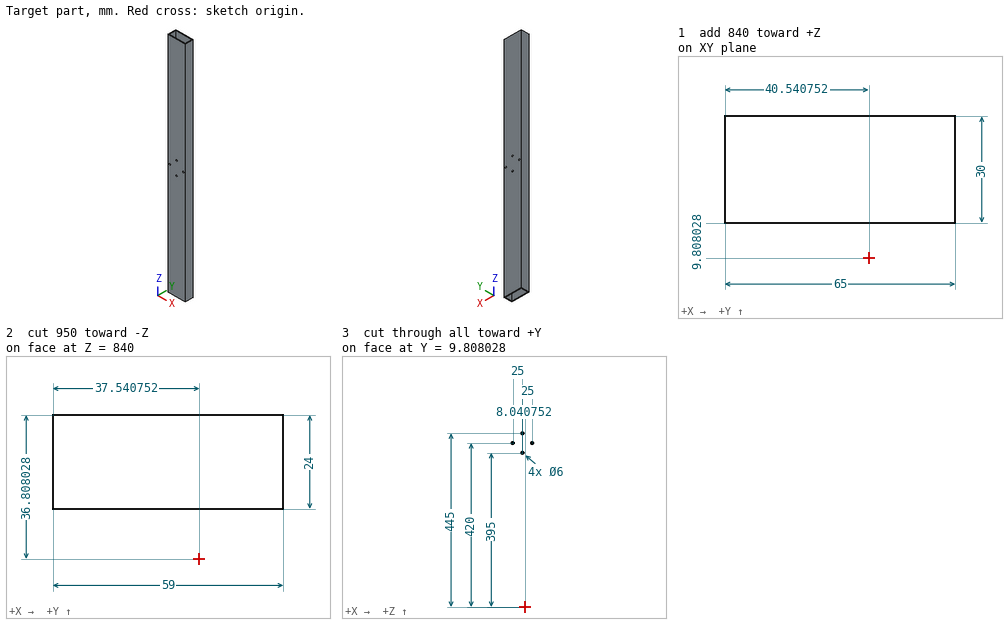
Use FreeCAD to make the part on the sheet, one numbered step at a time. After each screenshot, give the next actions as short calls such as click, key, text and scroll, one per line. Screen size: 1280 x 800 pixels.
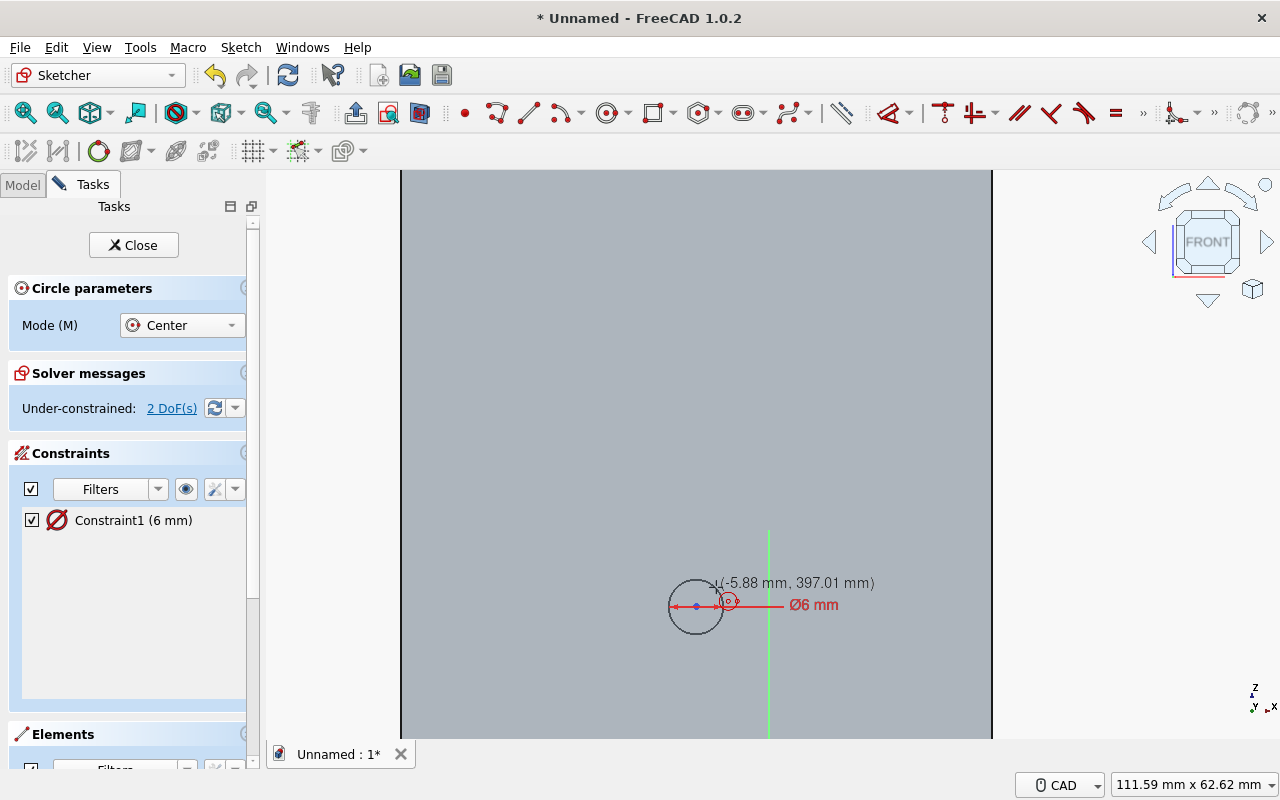
click(469, 379)
move(488, 360)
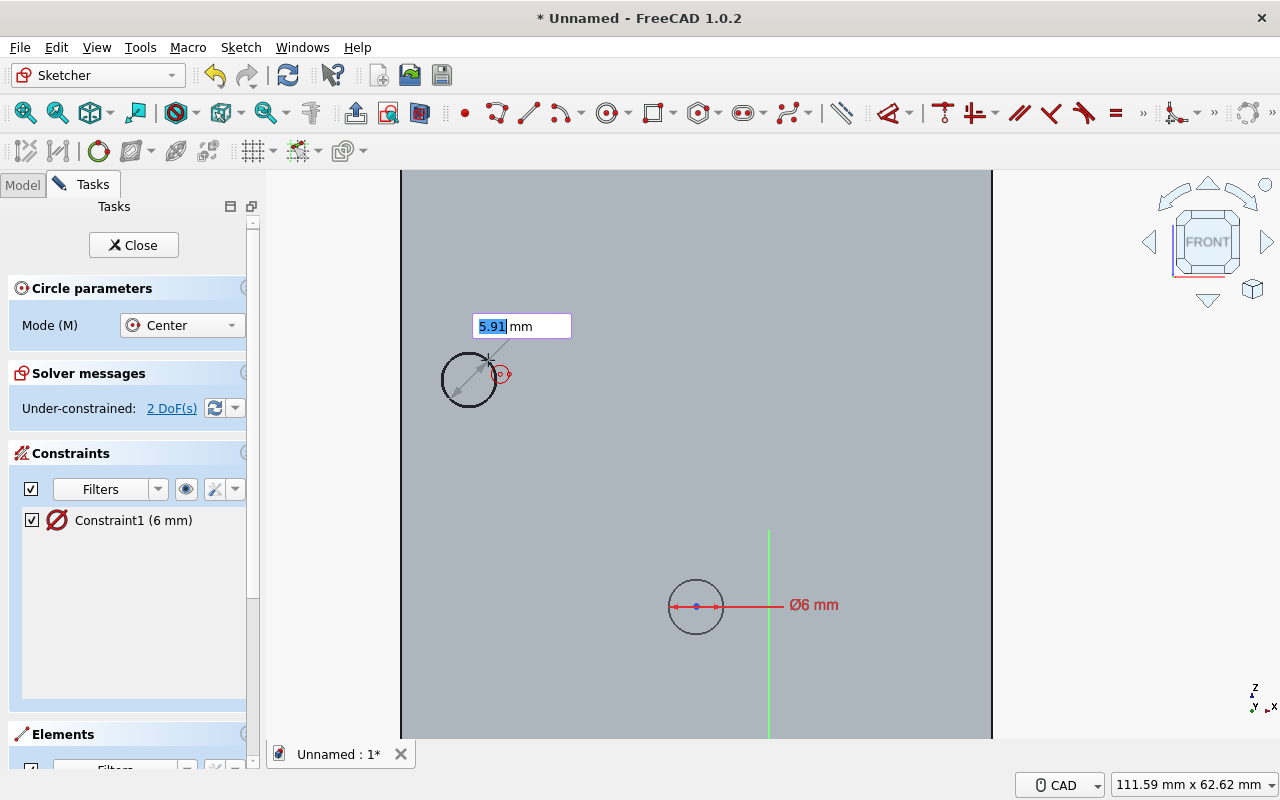
text(6)
key(Return)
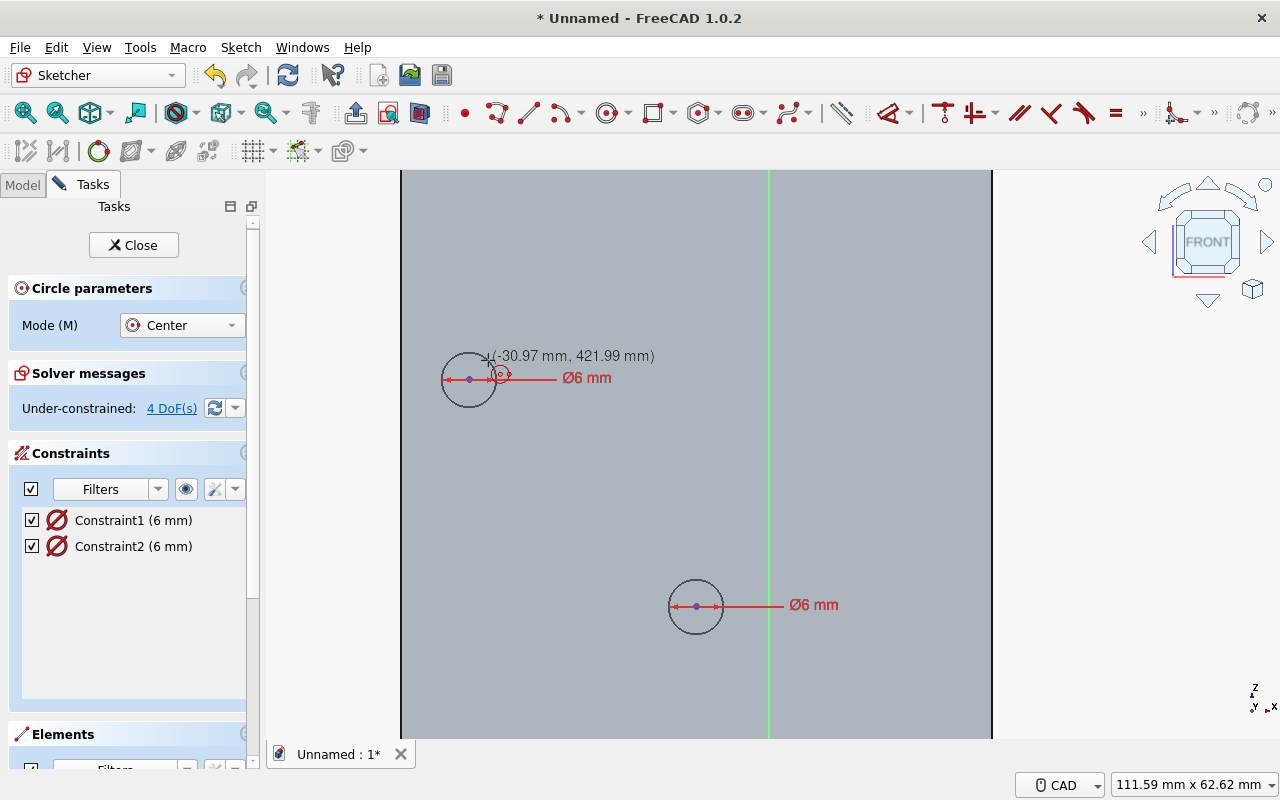
scroll(721, 608, down, 2)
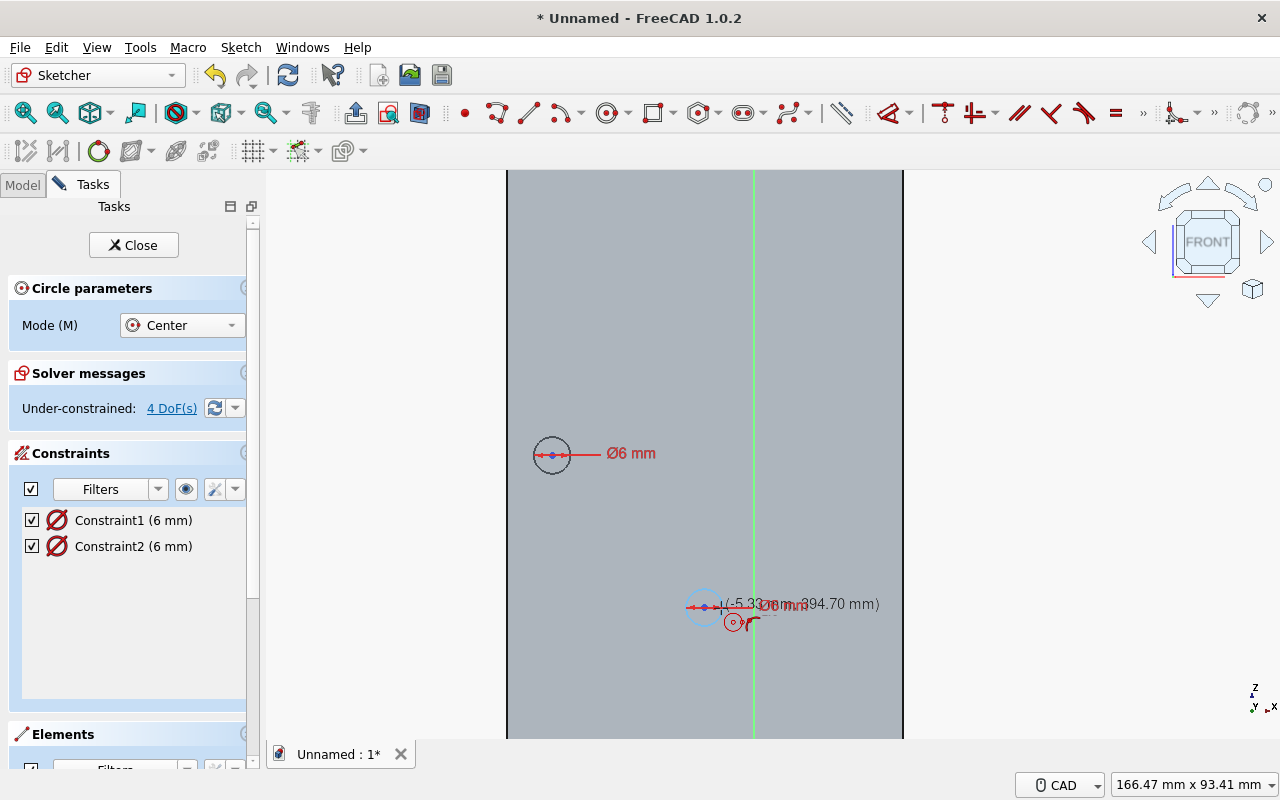
scroll(705, 303, up, 2)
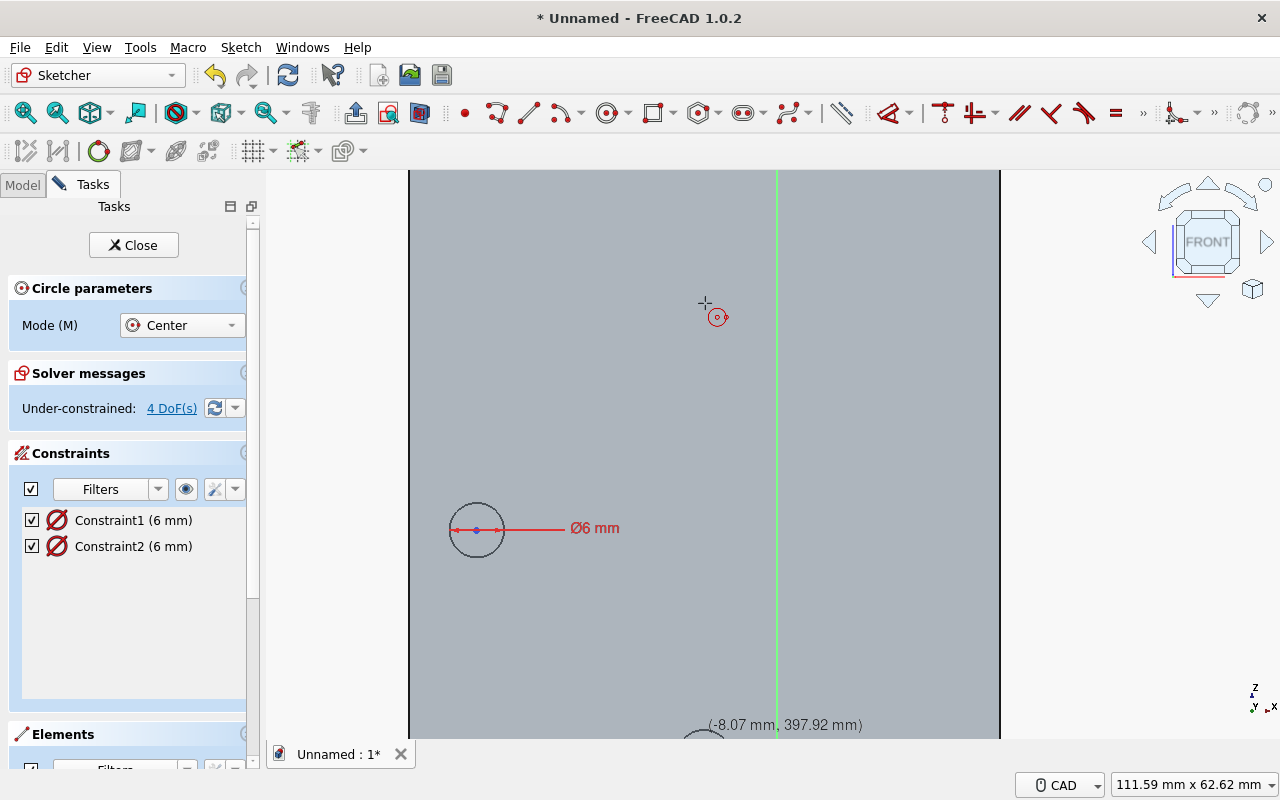
click(704, 302)
move(723, 283)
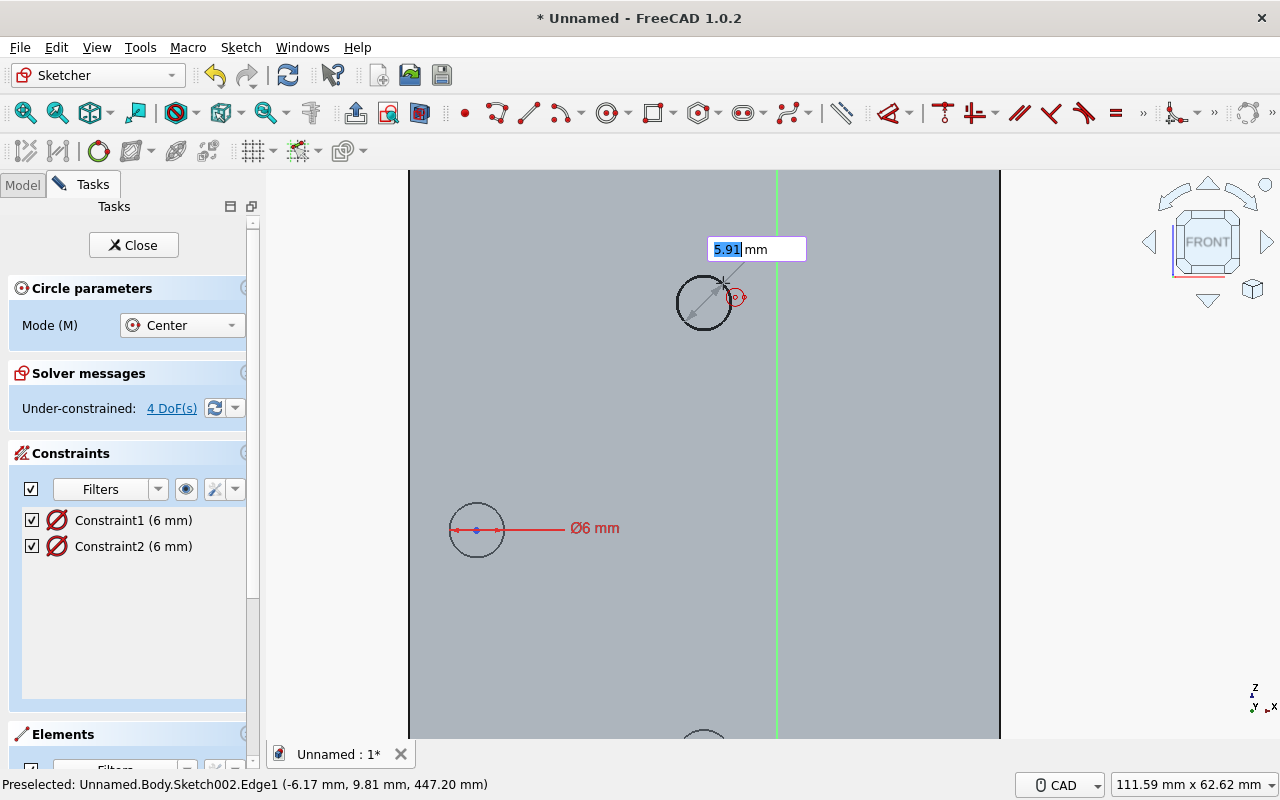
text(6)
key(Return)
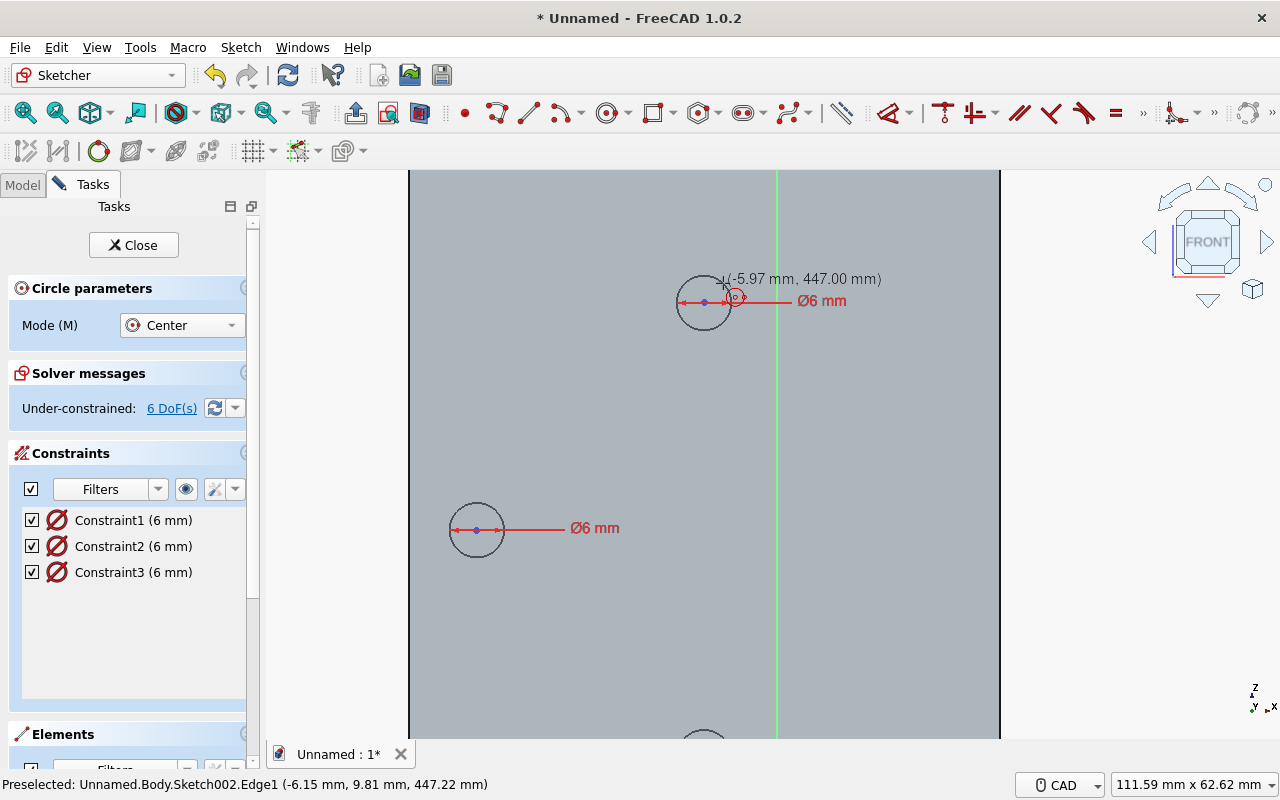
click(931, 529)
move(951, 510)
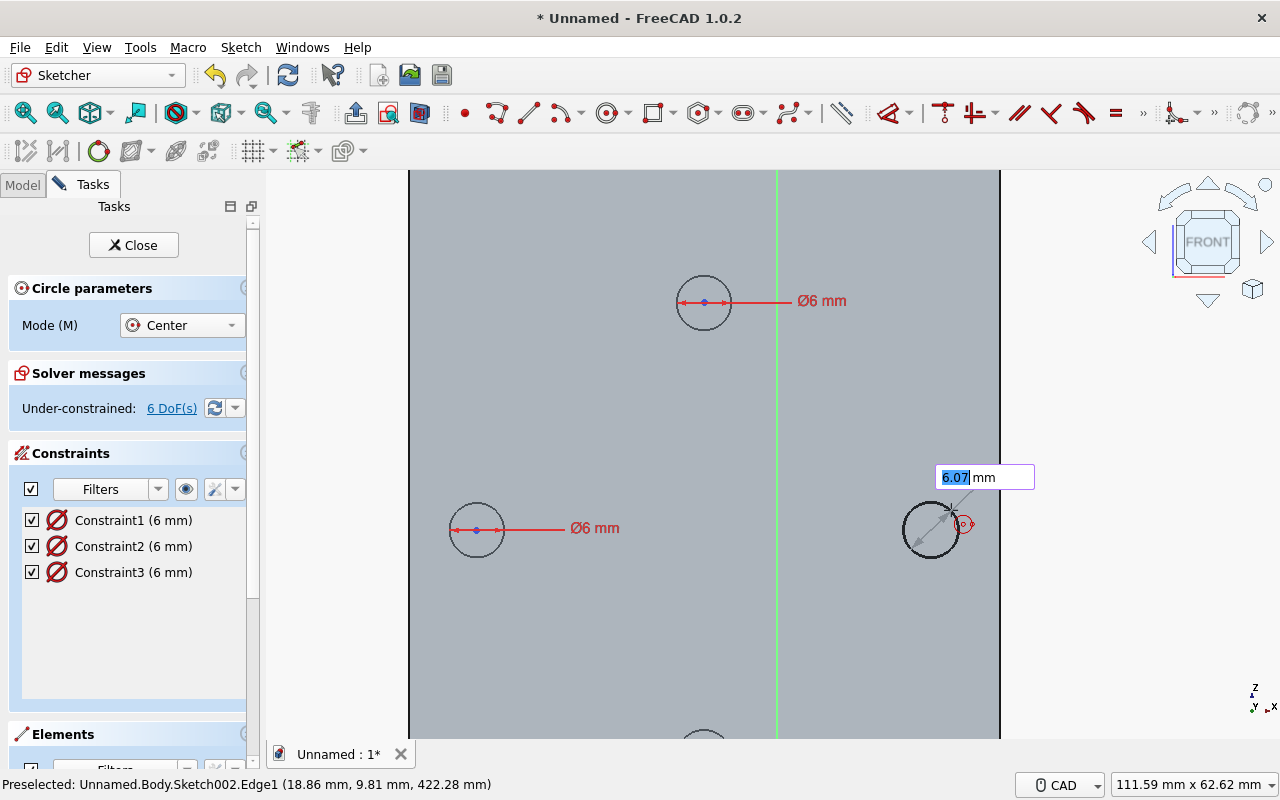
text(6)
key(Return)
key(Escape)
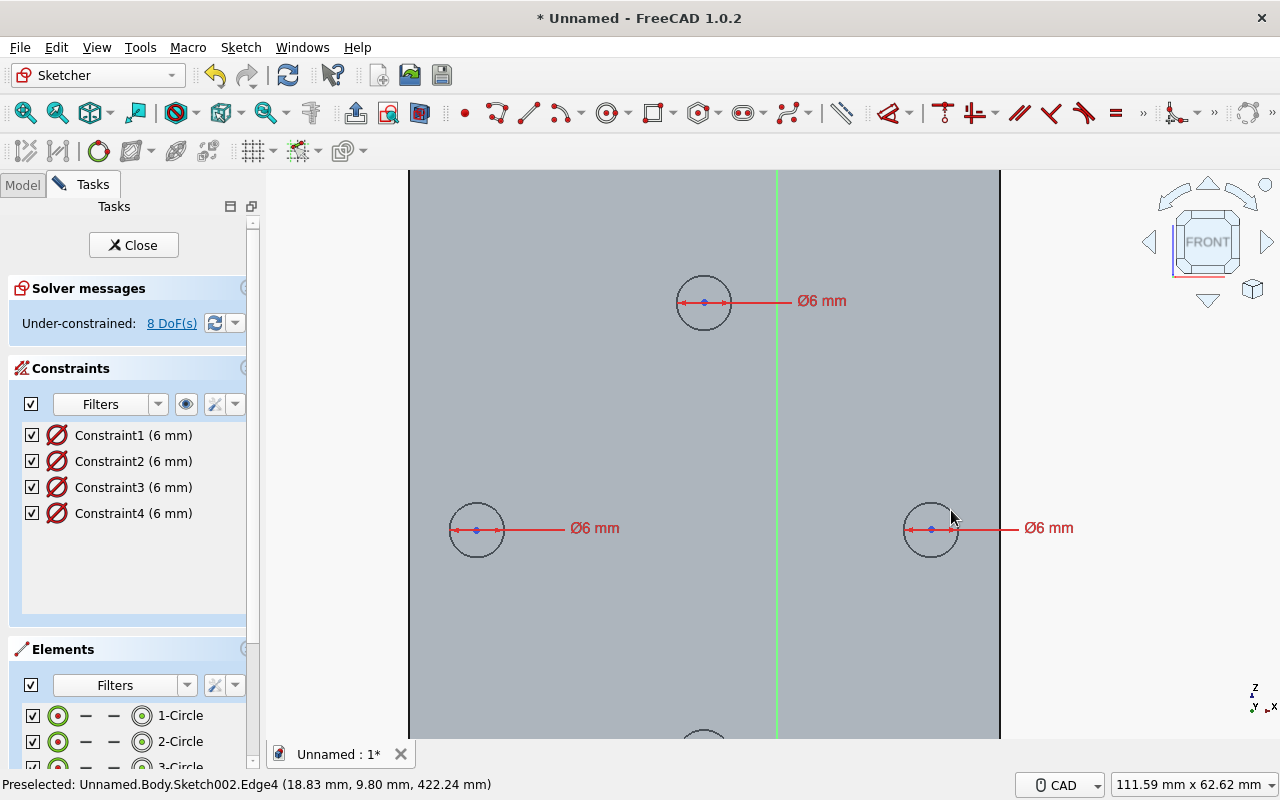
scroll(705, 302, down, 2)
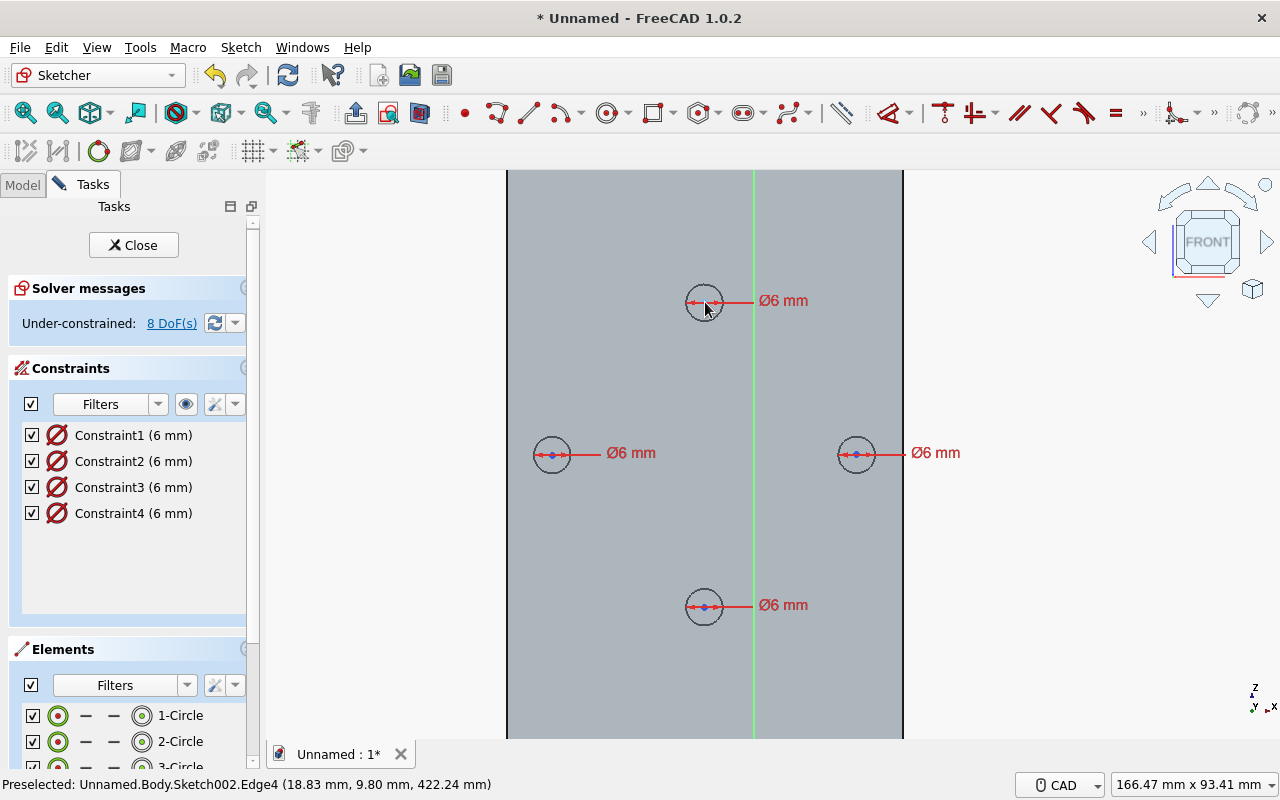
click(704, 607)